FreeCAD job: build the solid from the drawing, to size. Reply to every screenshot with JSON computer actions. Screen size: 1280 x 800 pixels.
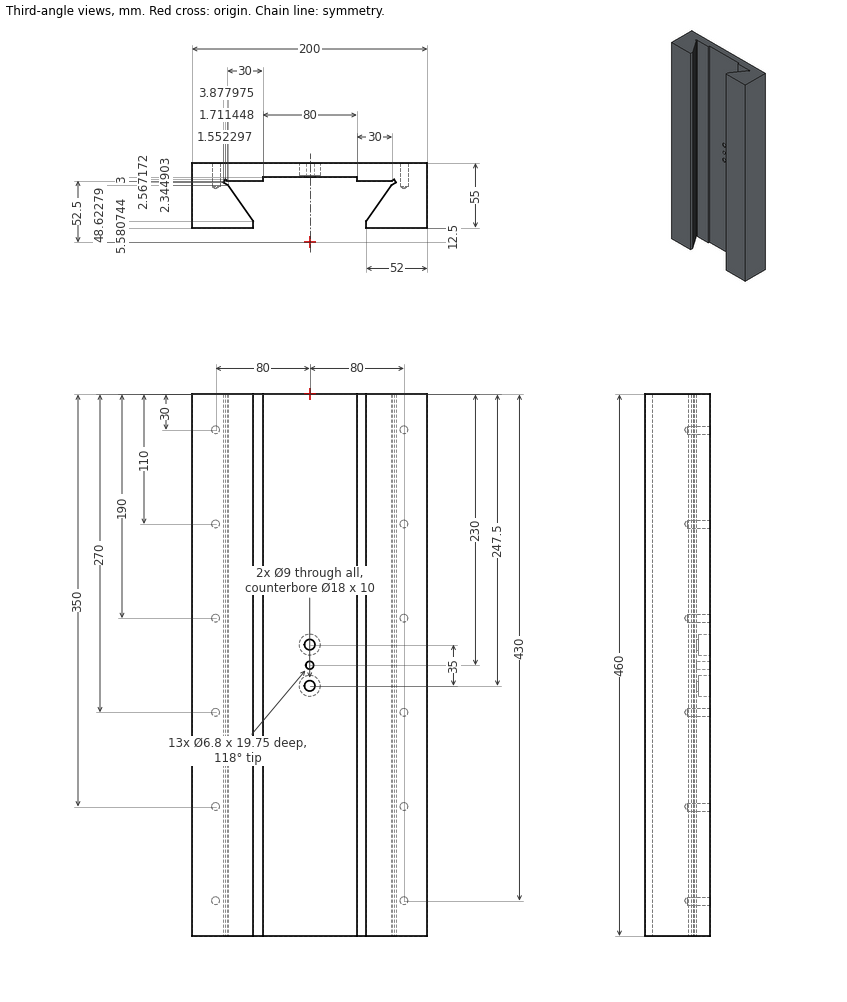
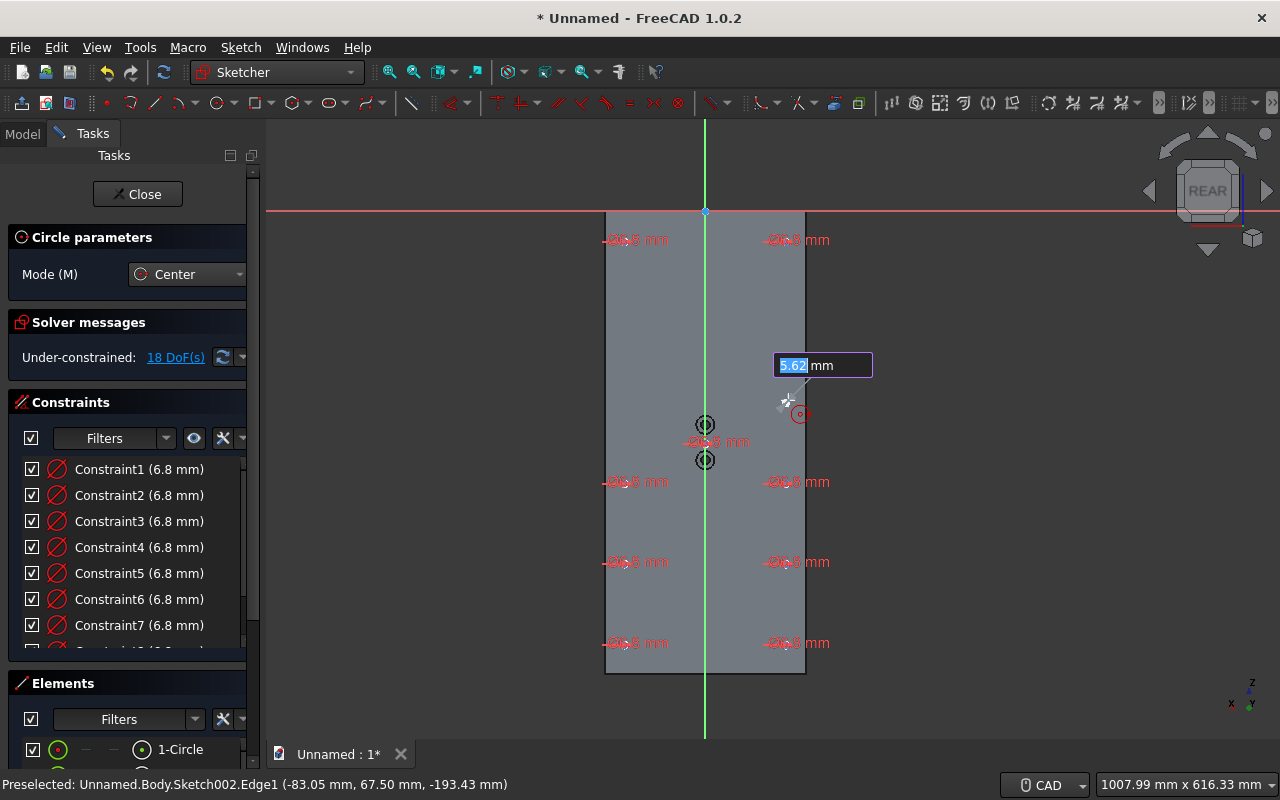
{"action": "type", "text": "6.8"}
{"action": "key", "text": "Return"}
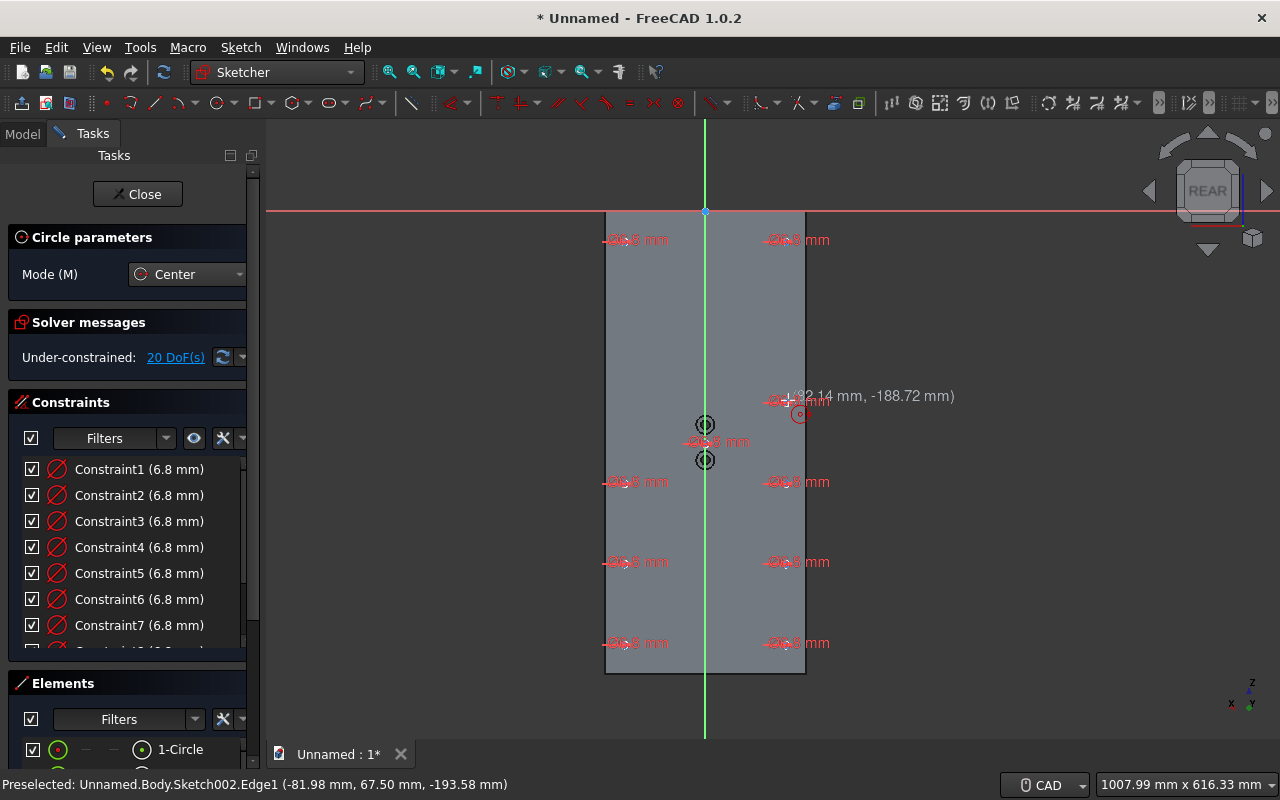
{"action": "scroll", "coordinate": [625, 402], "scroll_direction": "up", "scroll_amount": 10}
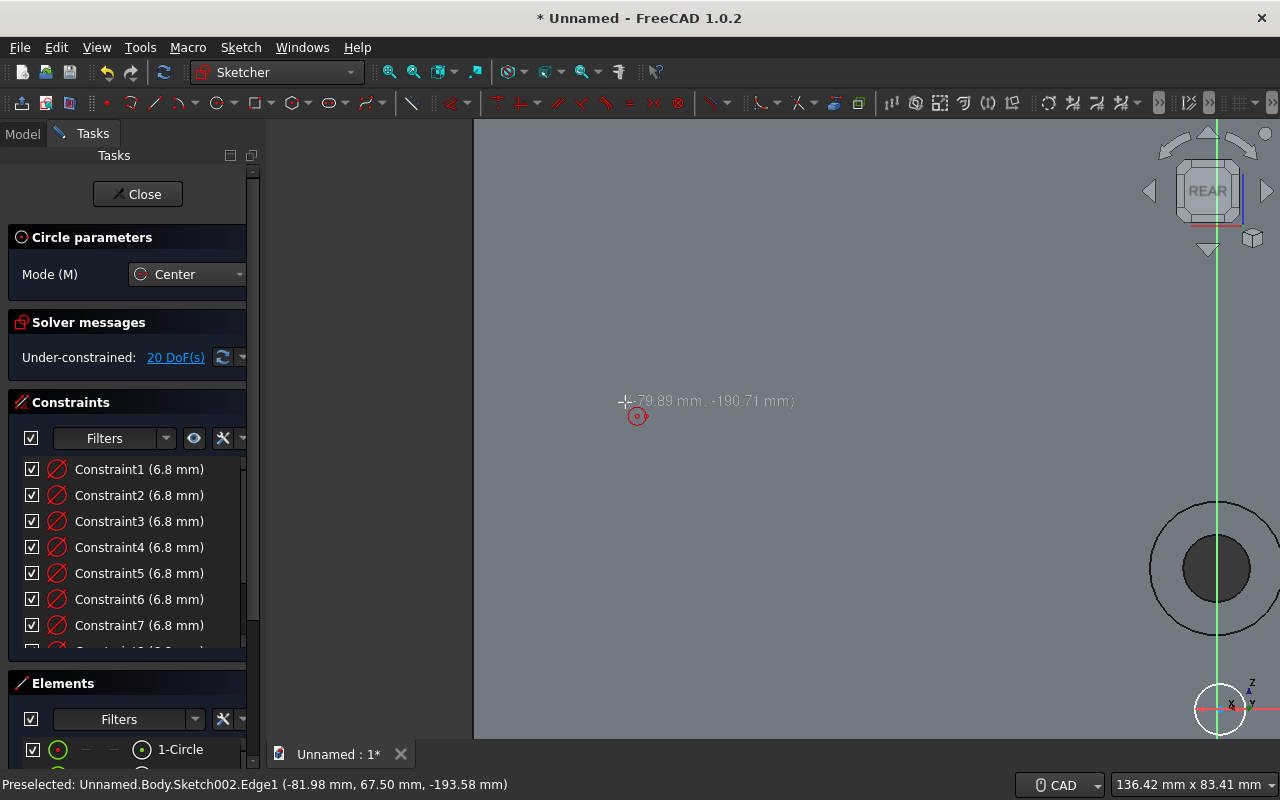
{"action": "scroll", "coordinate": [624, 402], "scroll_direction": "down", "scroll_amount": 10}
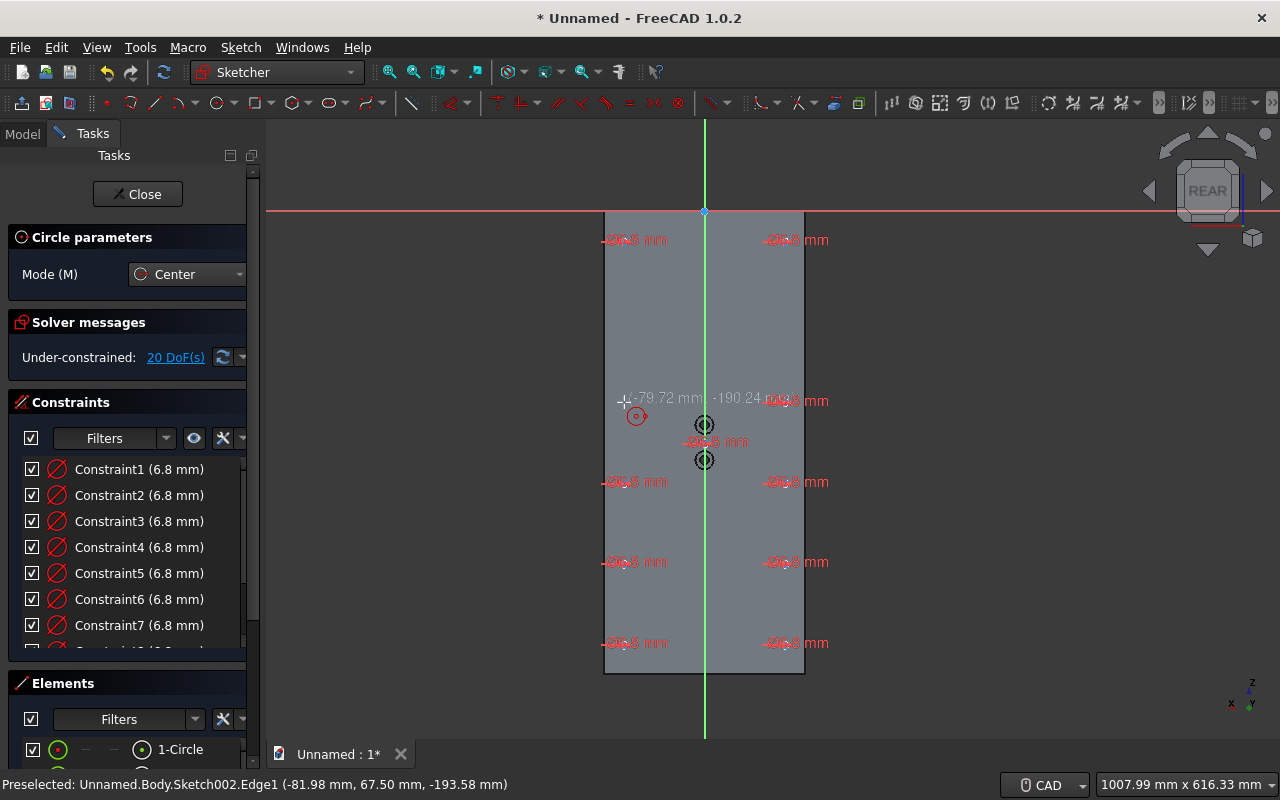
{"action": "left_click", "coordinate": [624, 402]}
{"action": "mouse_move", "coordinate": [626, 400]}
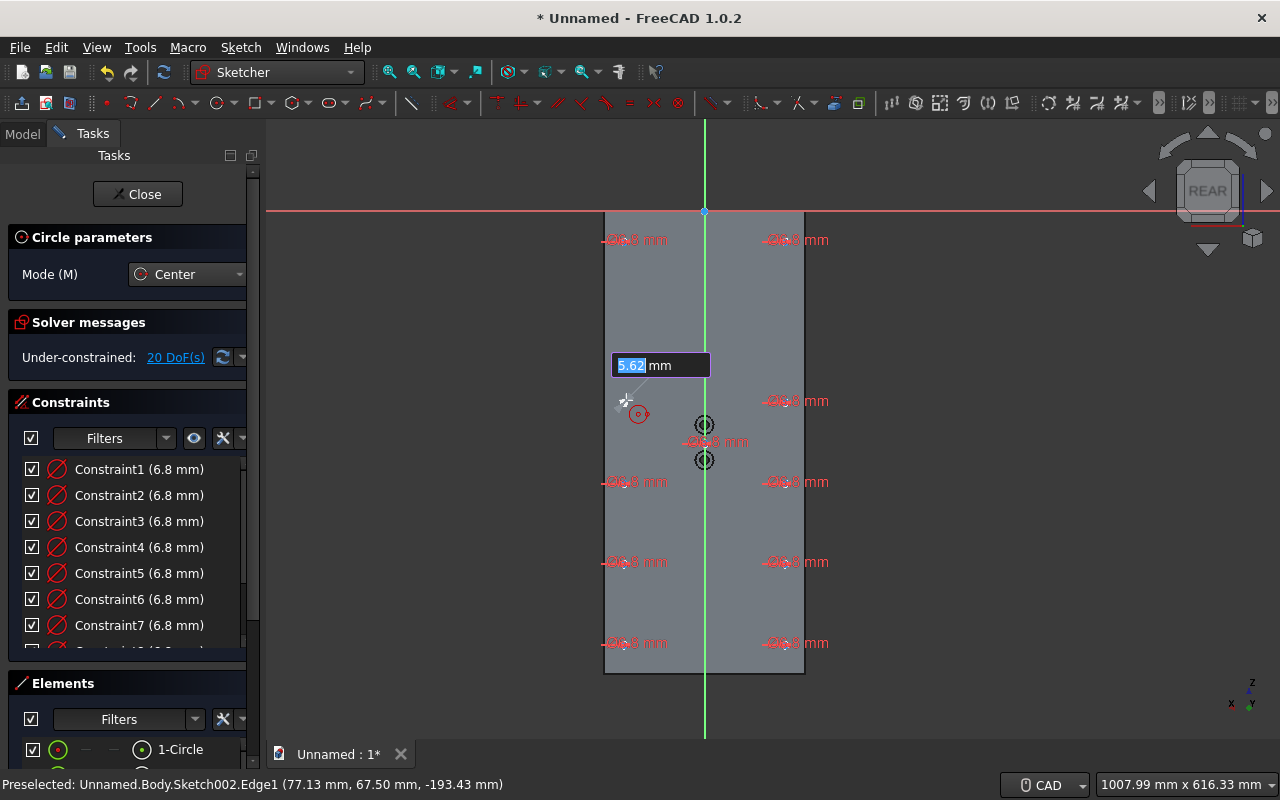
{"action": "type", "text": "6.8"}
{"action": "key", "text": "Return"}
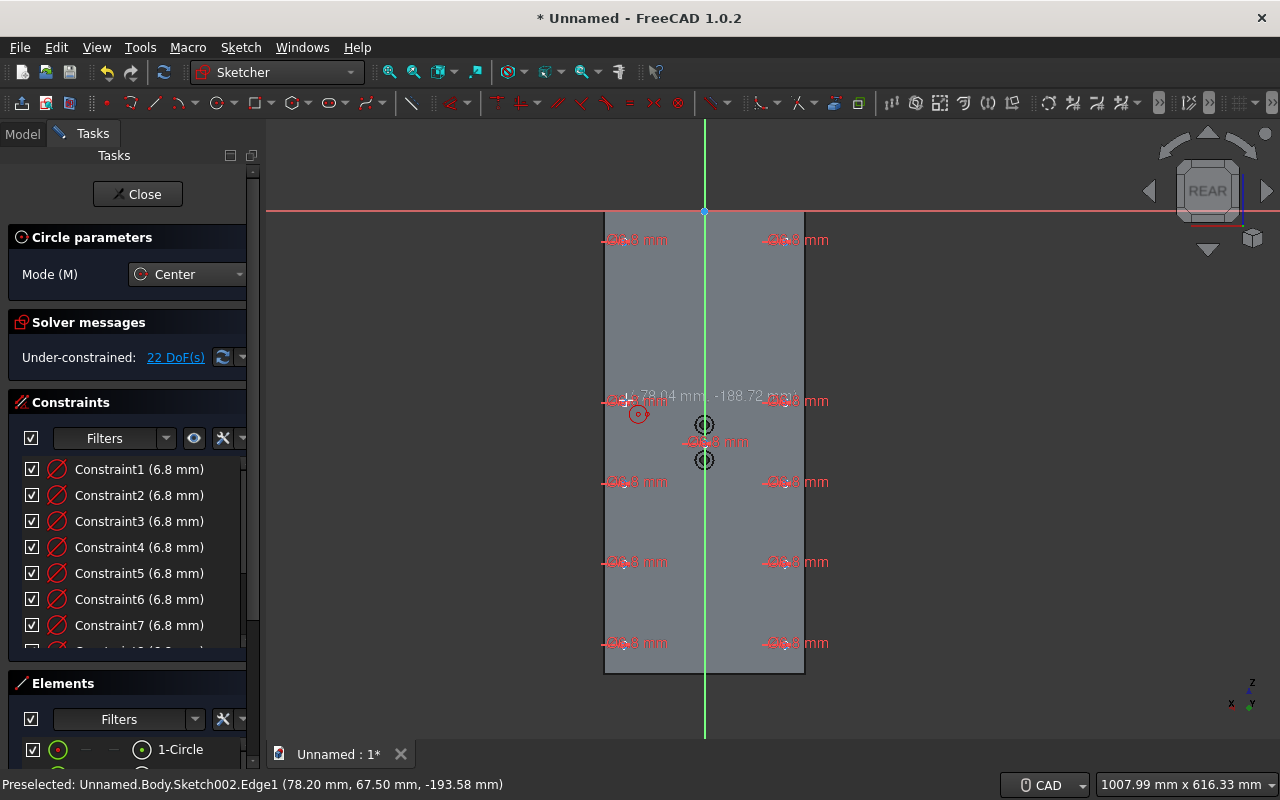
{"action": "scroll", "coordinate": [785, 322], "scroll_direction": "up", "scroll_amount": 10}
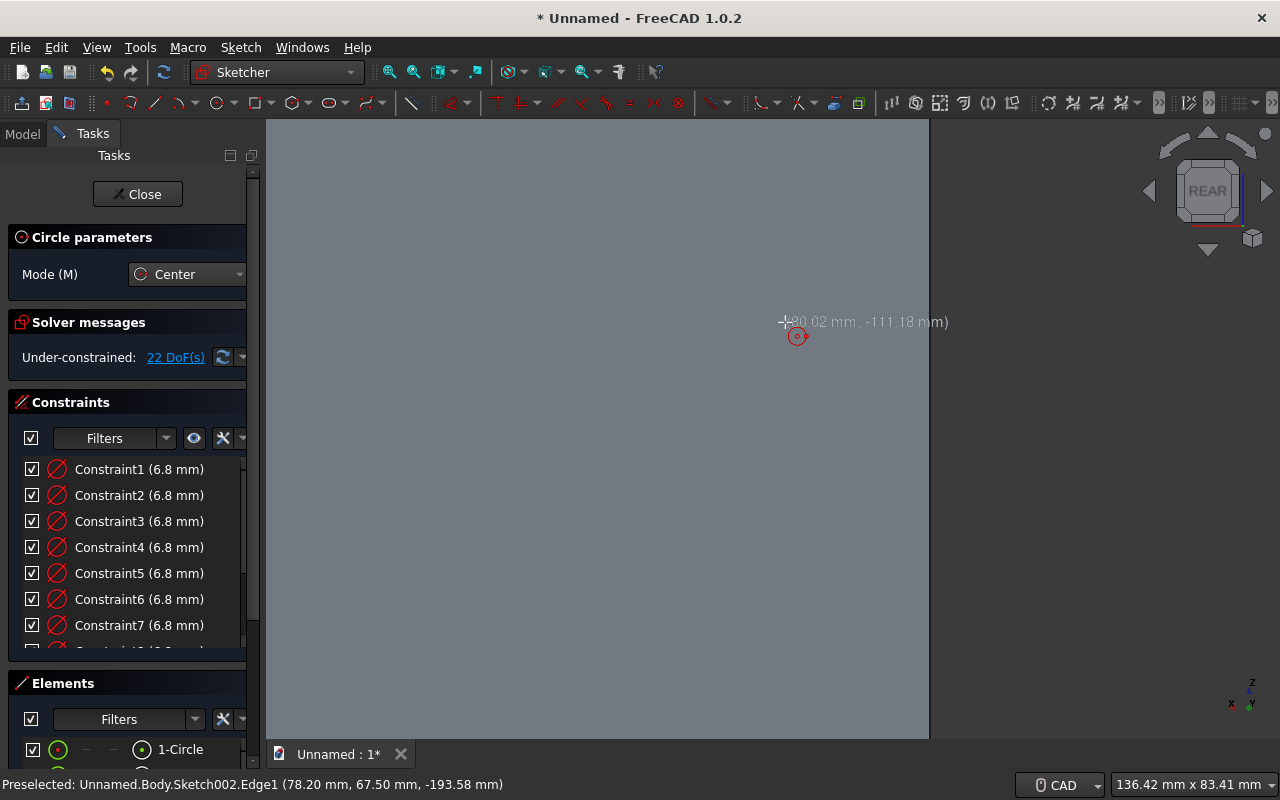
{"action": "scroll", "coordinate": [786, 322], "scroll_direction": "down", "scroll_amount": 10}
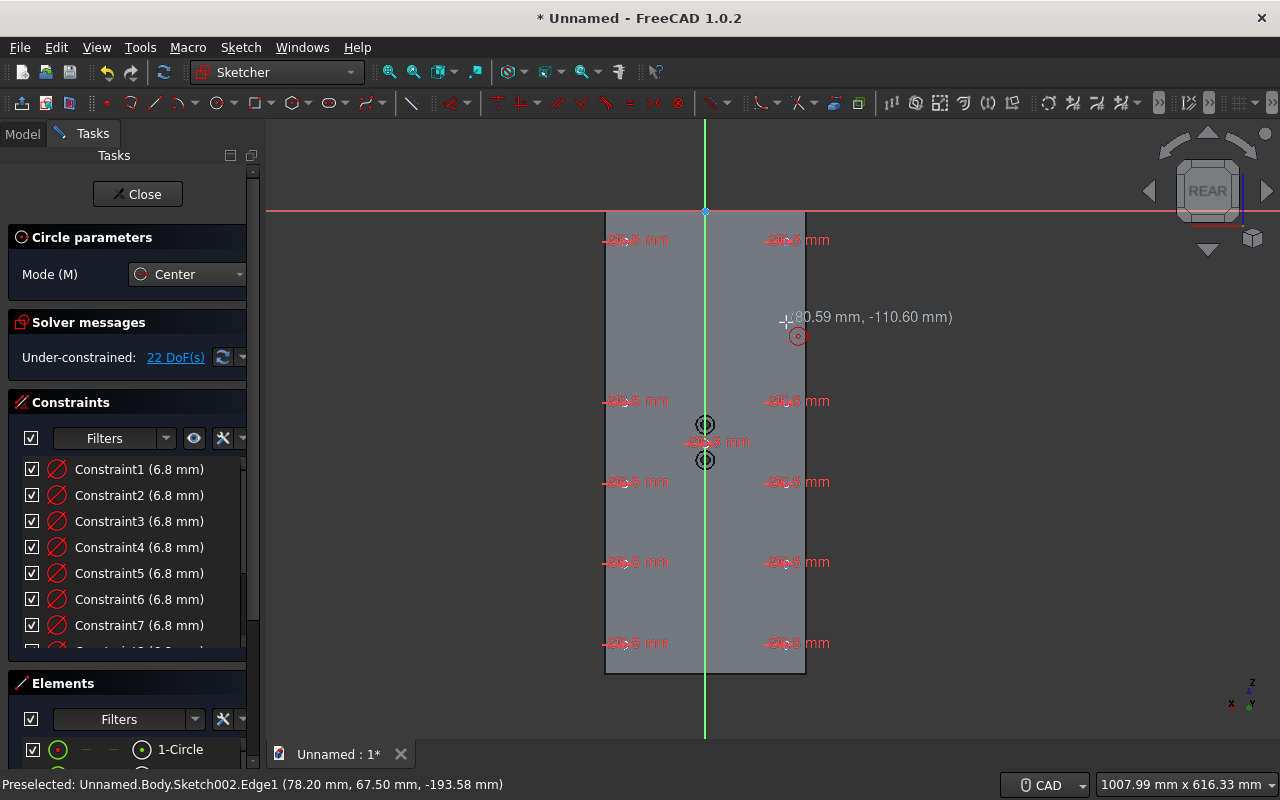
{"action": "left_click", "coordinate": [786, 322]}
{"action": "mouse_move", "coordinate": [788, 319]}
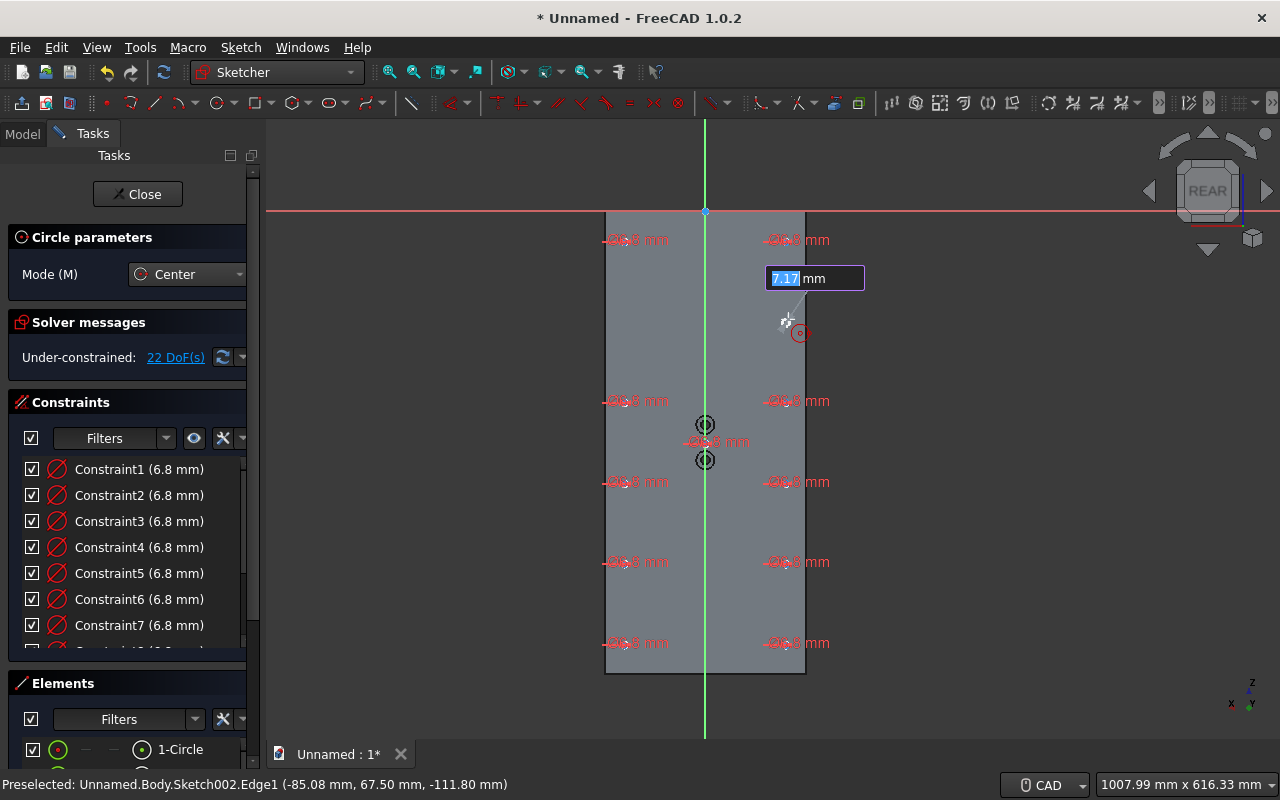
{"action": "type", "text": "6.8"}
{"action": "key", "text": "Return"}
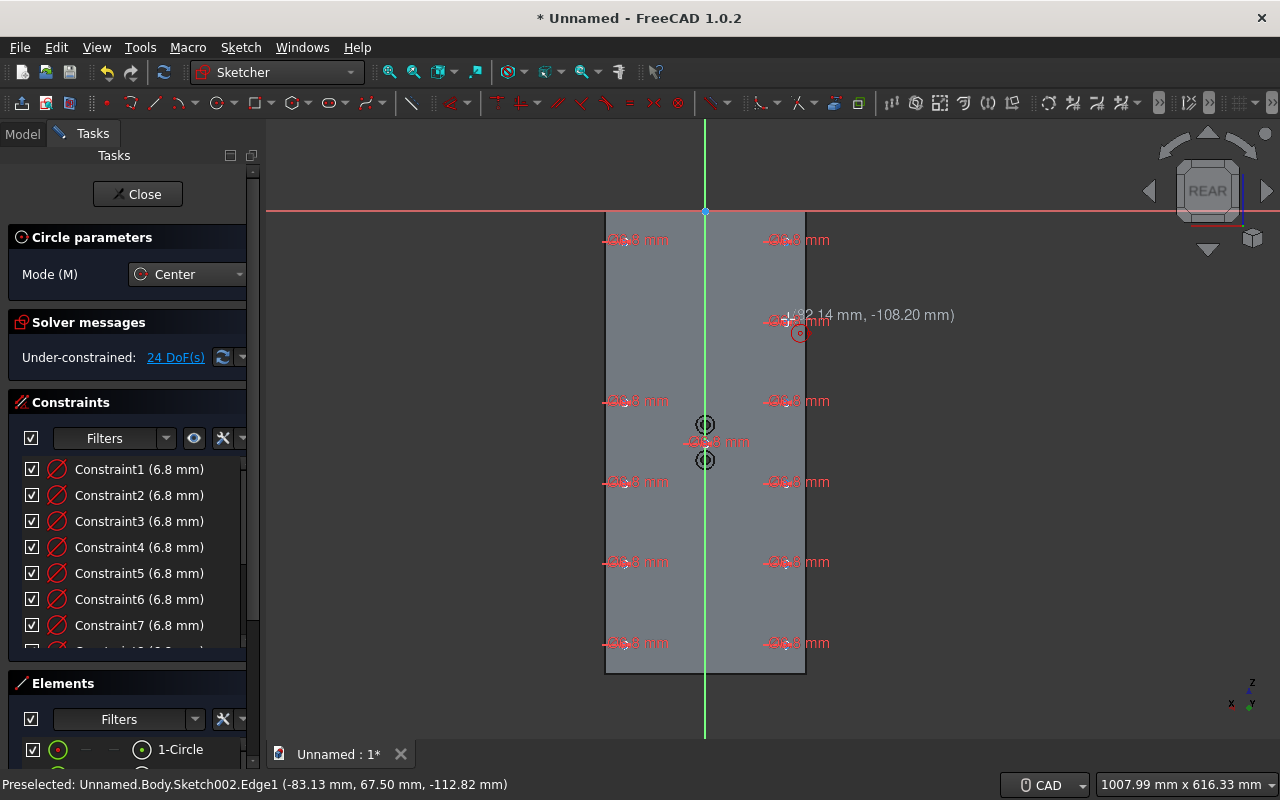
{"action": "scroll", "coordinate": [625, 322], "scroll_direction": "up", "scroll_amount": 10}